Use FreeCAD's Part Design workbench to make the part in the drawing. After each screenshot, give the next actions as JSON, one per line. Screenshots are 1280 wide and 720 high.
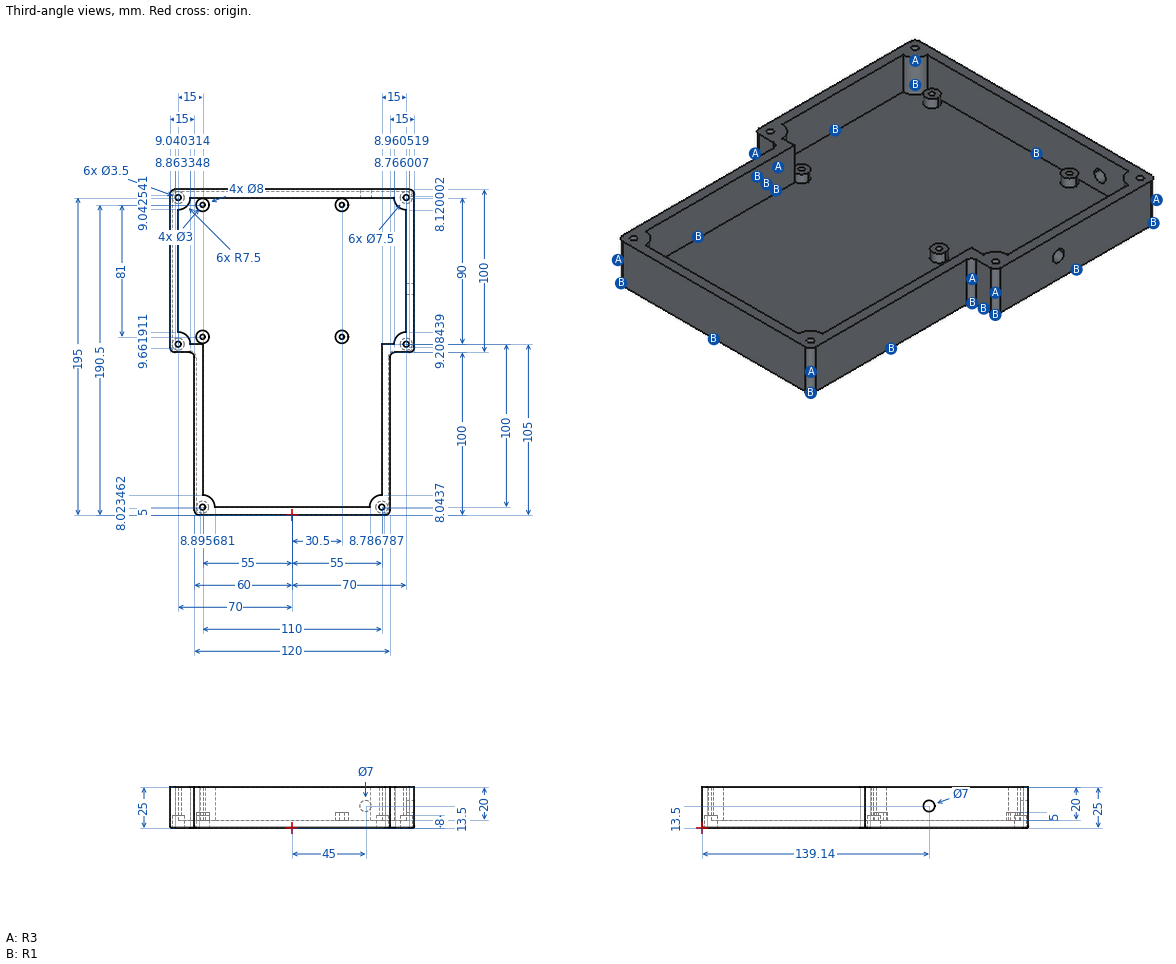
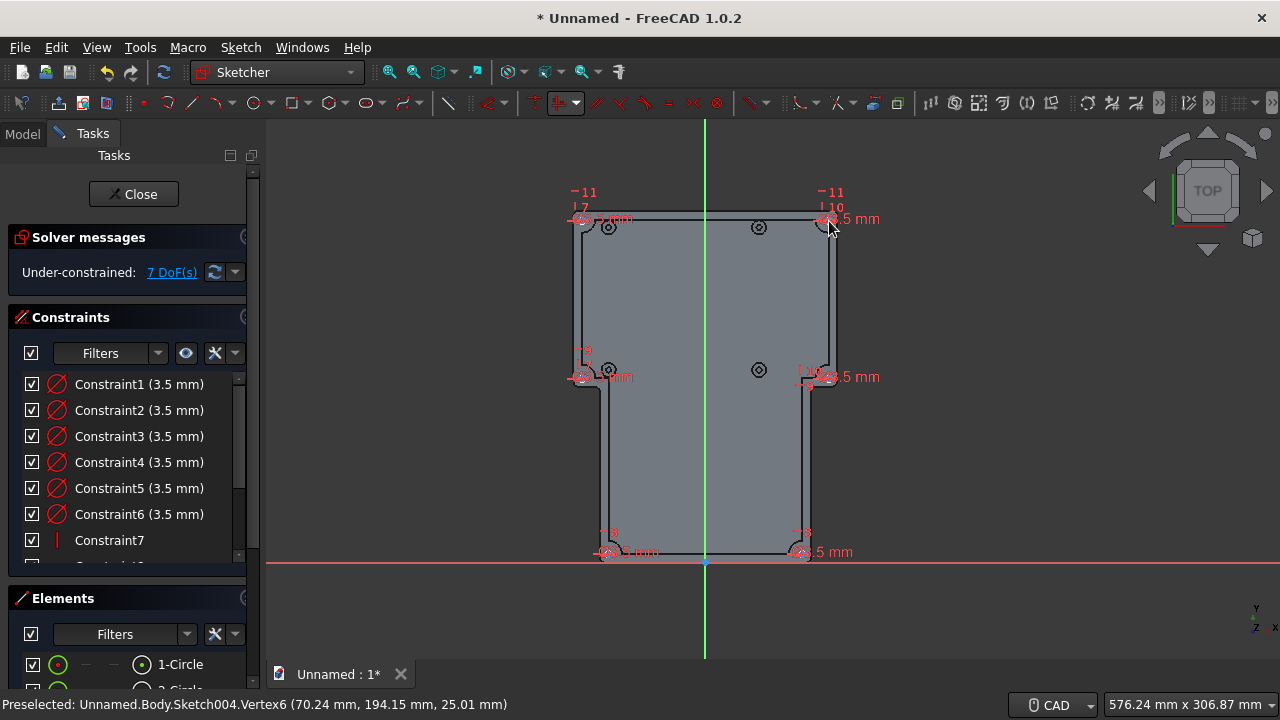
{"action": "key", "text": "d"}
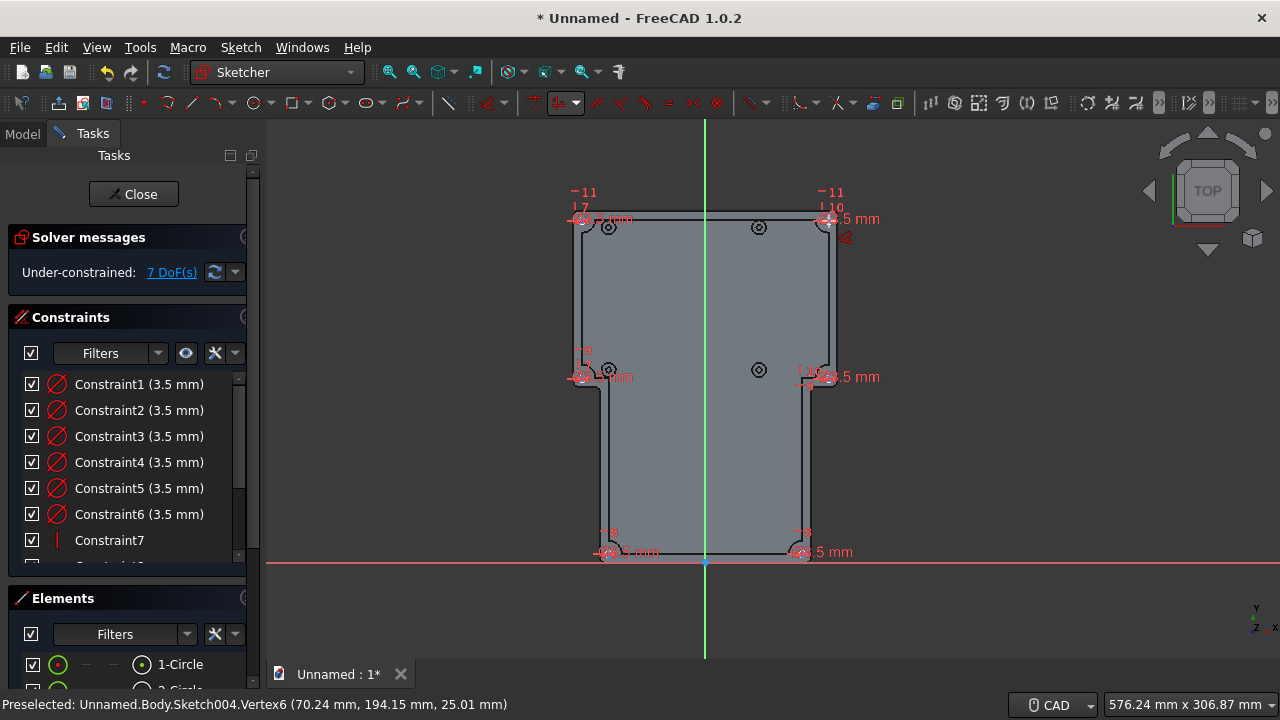
{"action": "scroll", "coordinate": [608, 554], "scroll_direction": "up", "scroll_amount": 8}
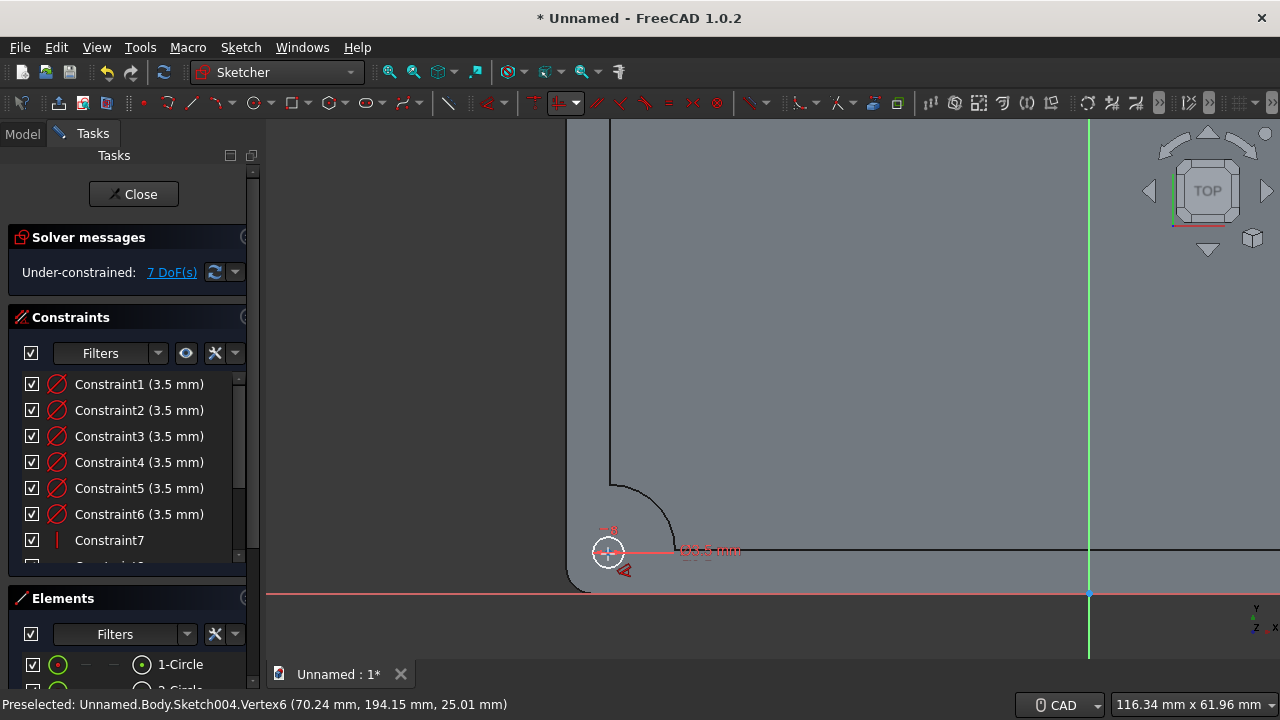
{"action": "left_click", "coordinate": [608, 553]}
{"action": "left_click", "coordinate": [574, 573]}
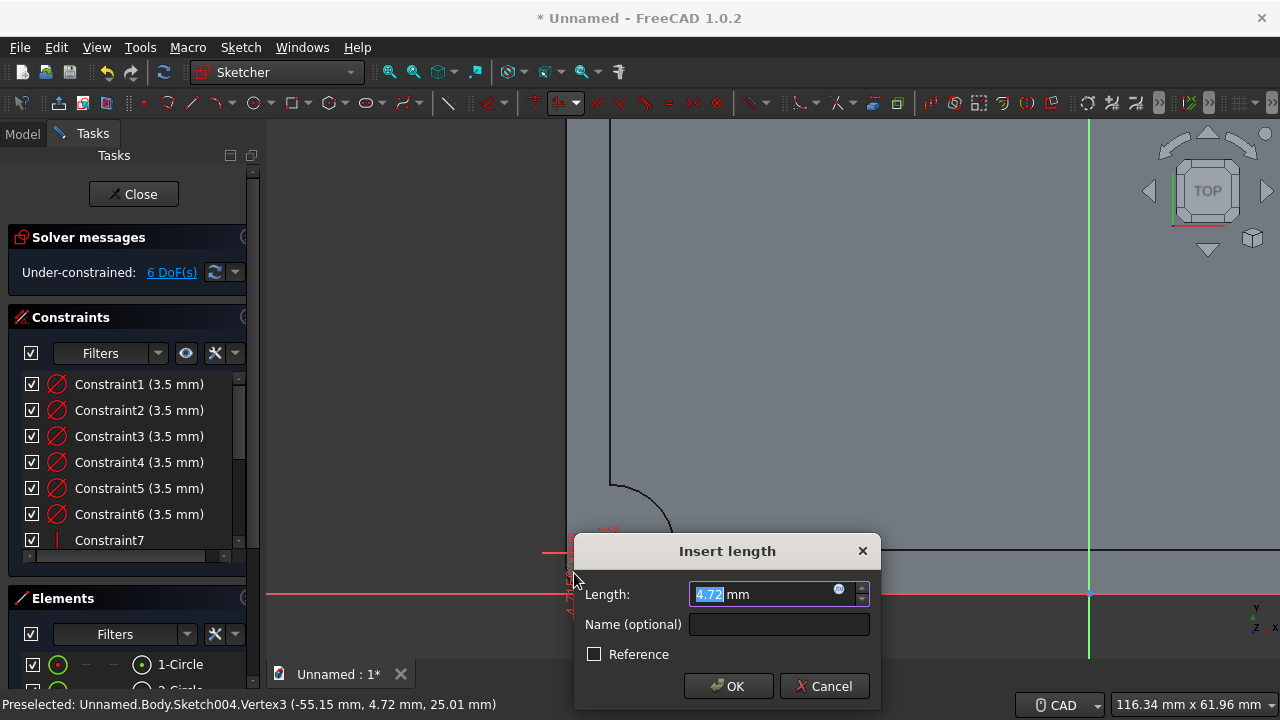
{"action": "type", "text": "5"}
{"action": "key", "text": "Return"}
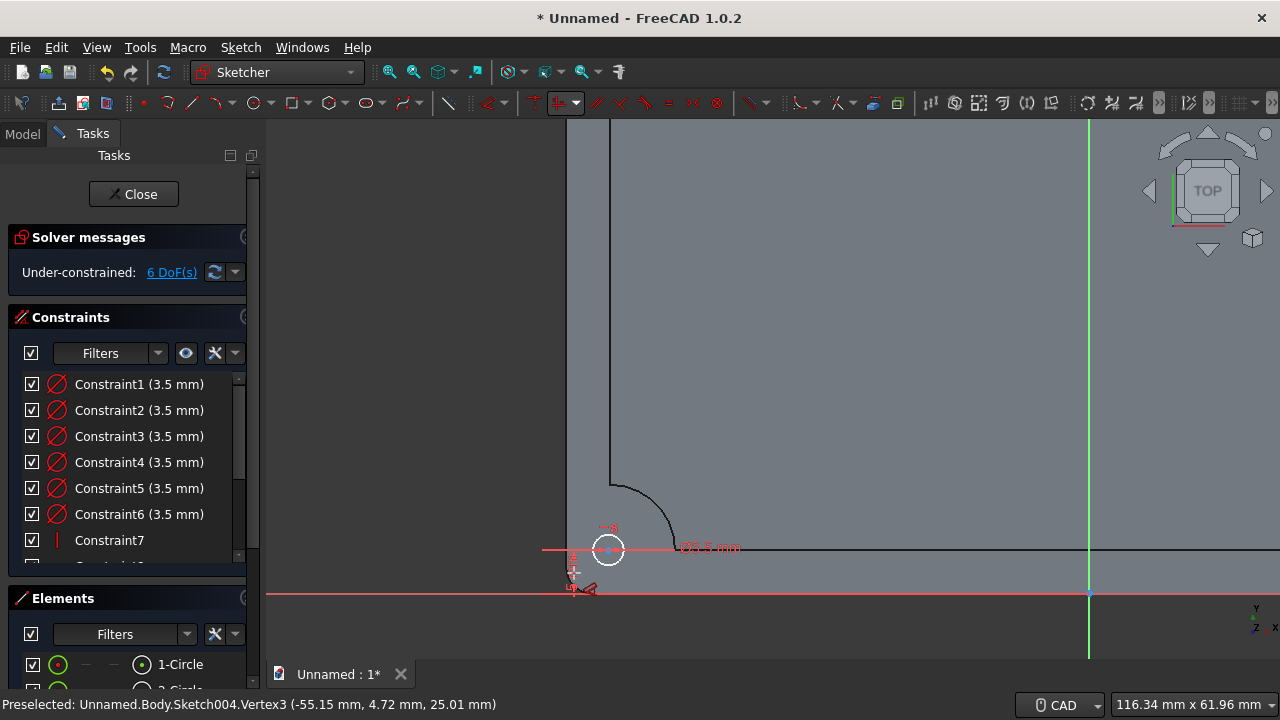
{"action": "scroll", "coordinate": [607, 554], "scroll_direction": "down", "scroll_amount": 8}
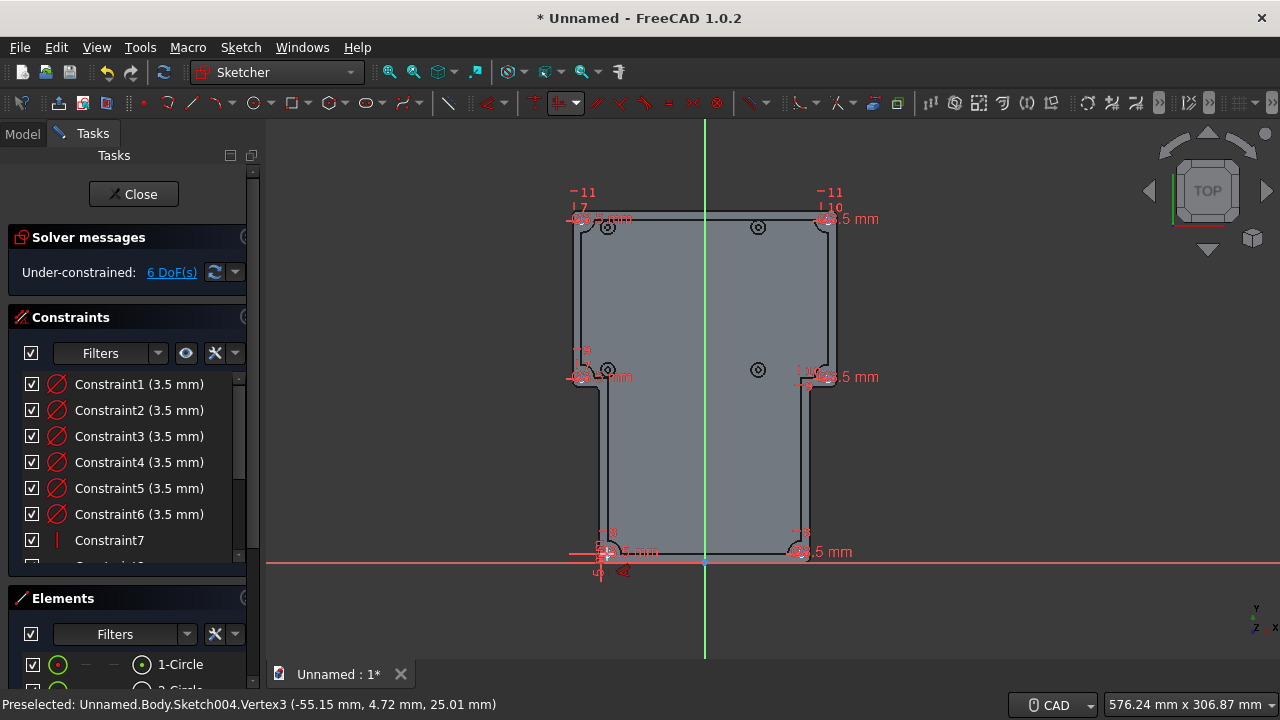
{"action": "left_click", "coordinate": [581, 221]}
{"action": "left_click", "coordinate": [643, 597]}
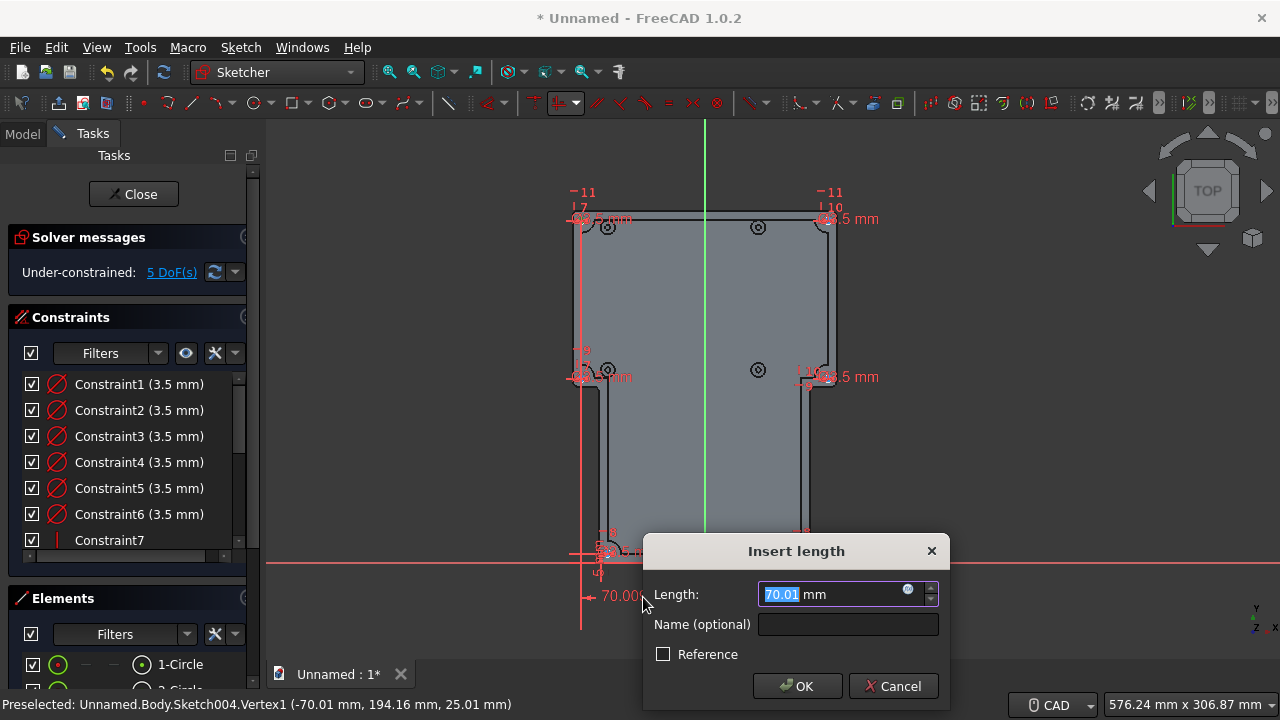
{"action": "type", "text": "70"}
{"action": "key", "text": "Return"}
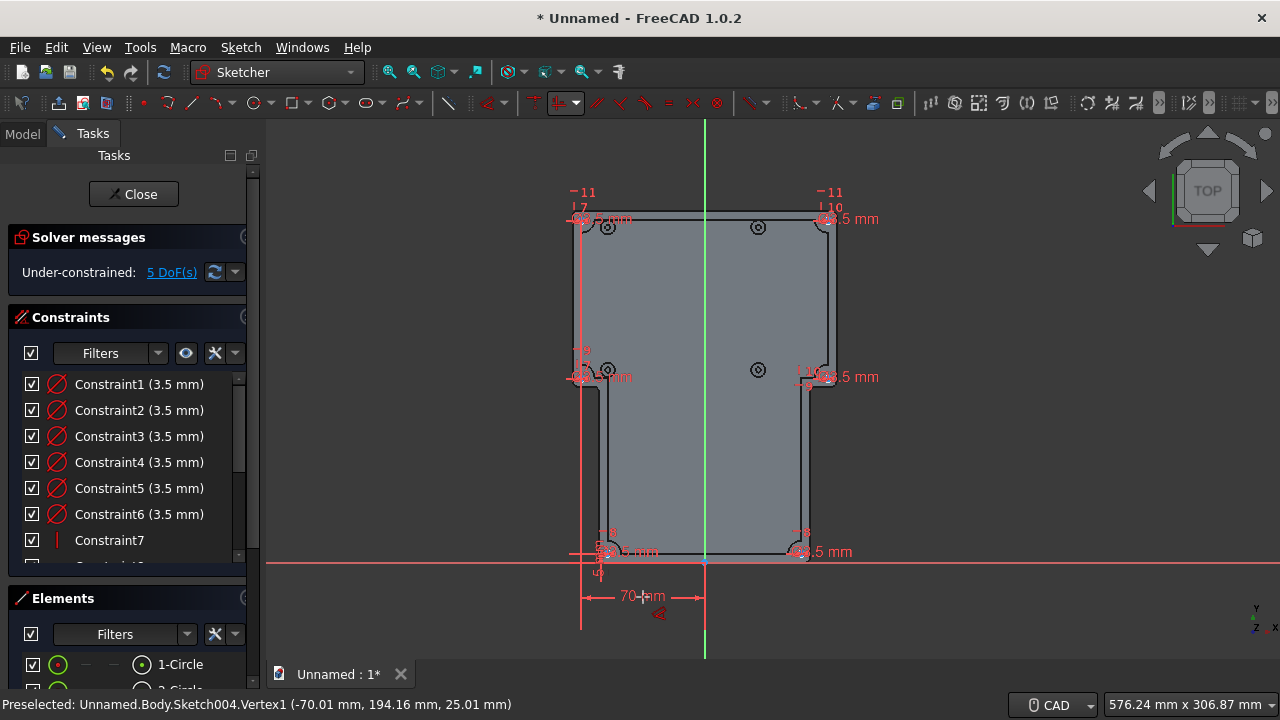
{"action": "left_click", "coordinate": [608, 554]}
{"action": "left_click", "coordinate": [656, 520]}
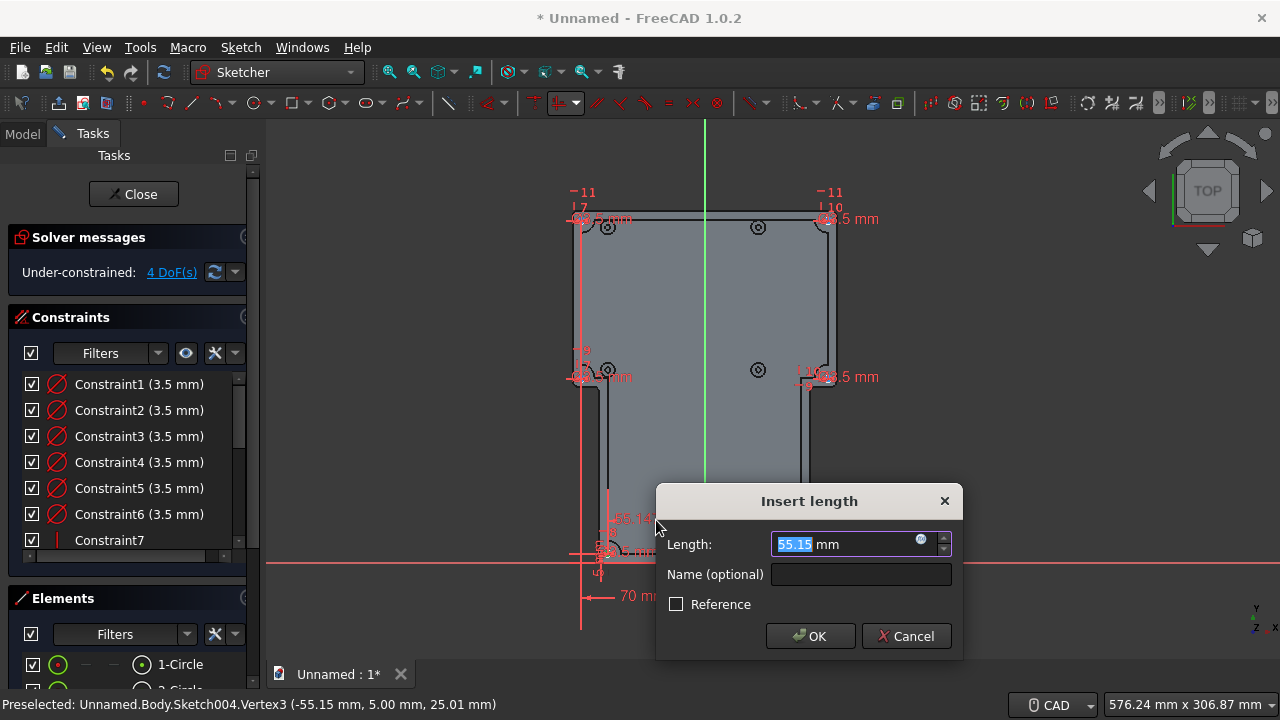
{"action": "type", "text": "55"}
{"action": "key", "text": "Return"}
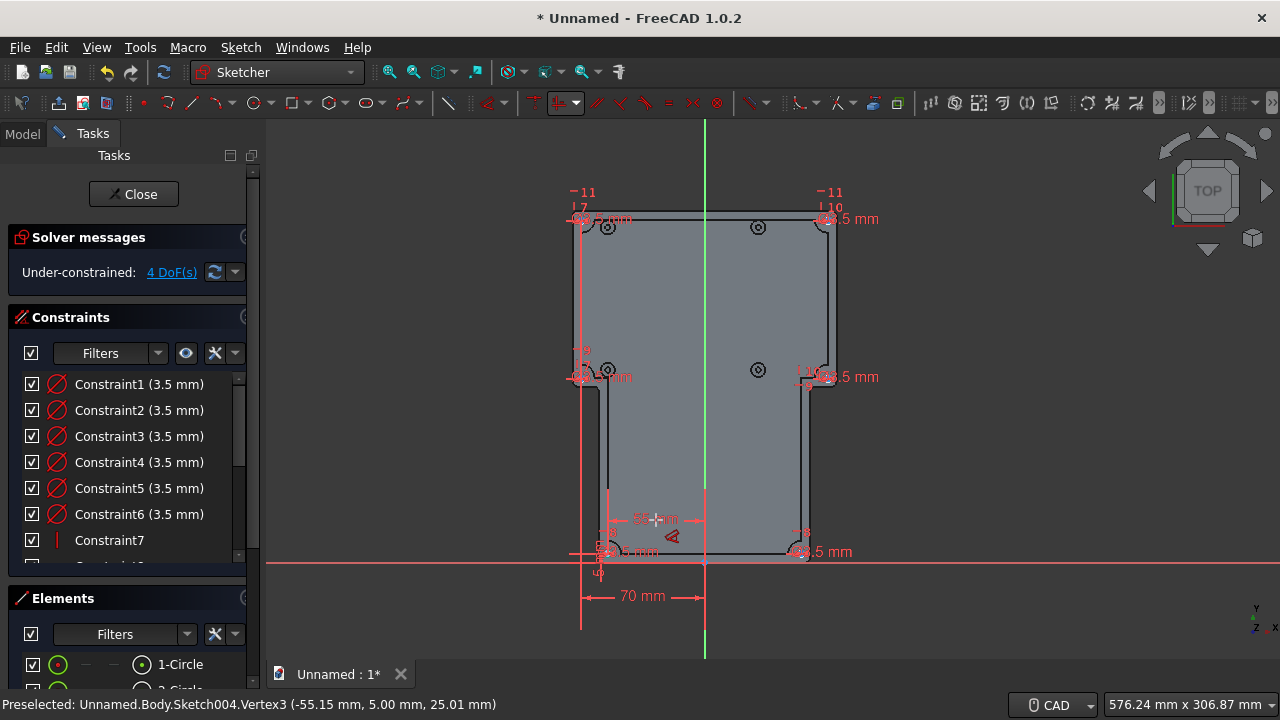
{"action": "left_click", "coordinate": [801, 554]}
{"action": "left_click", "coordinate": [753, 597]}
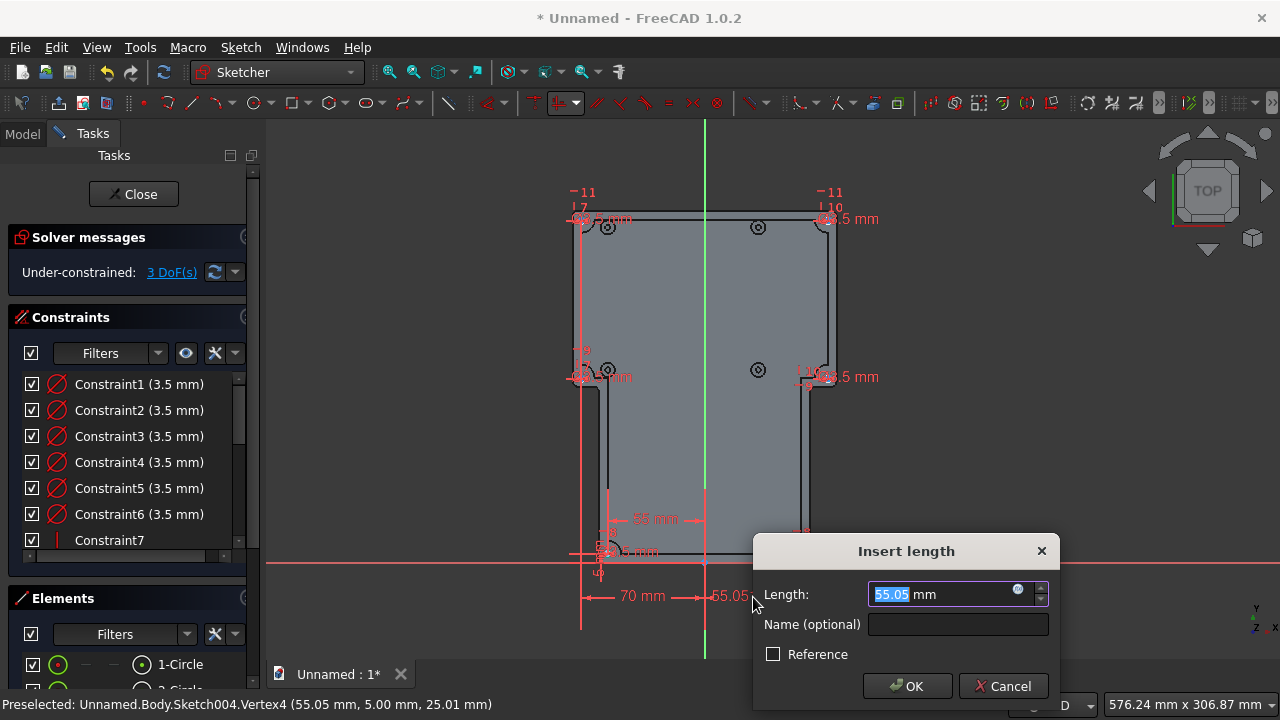
{"action": "type", "text": "55"}
{"action": "key", "text": "Return"}